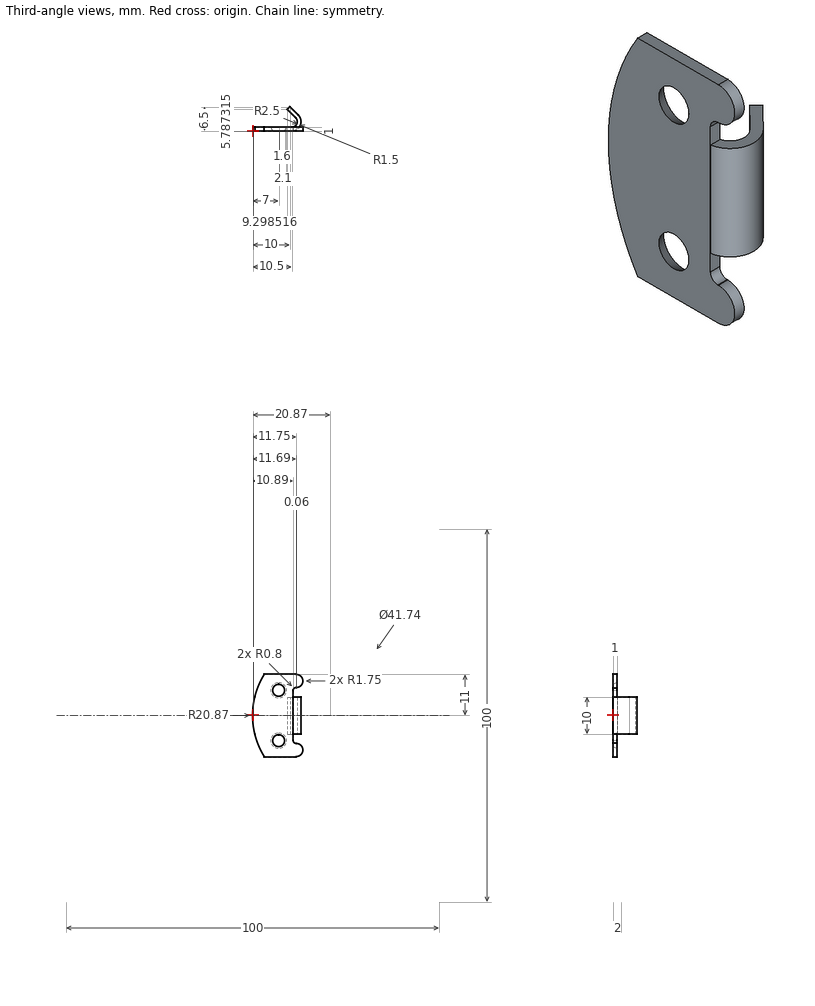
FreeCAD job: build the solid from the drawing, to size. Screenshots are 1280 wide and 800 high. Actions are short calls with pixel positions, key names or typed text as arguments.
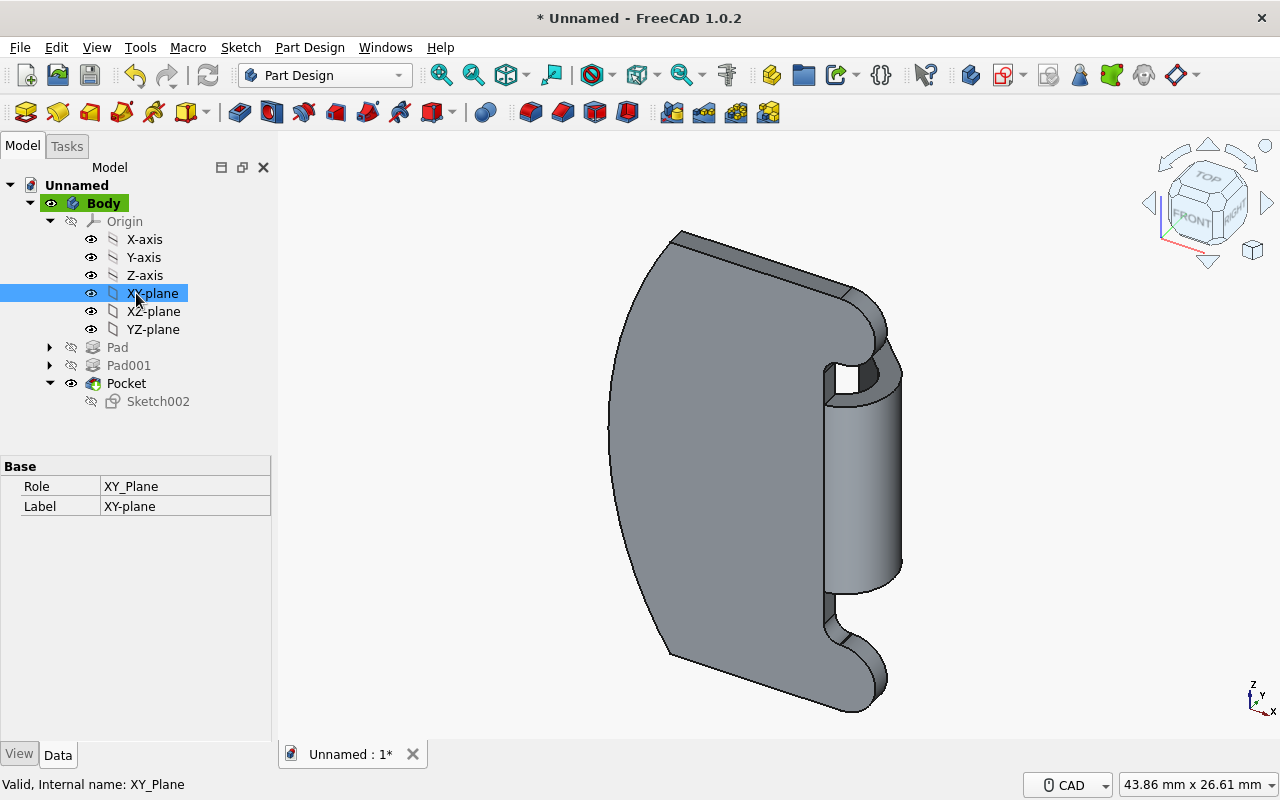
click(1176, 76)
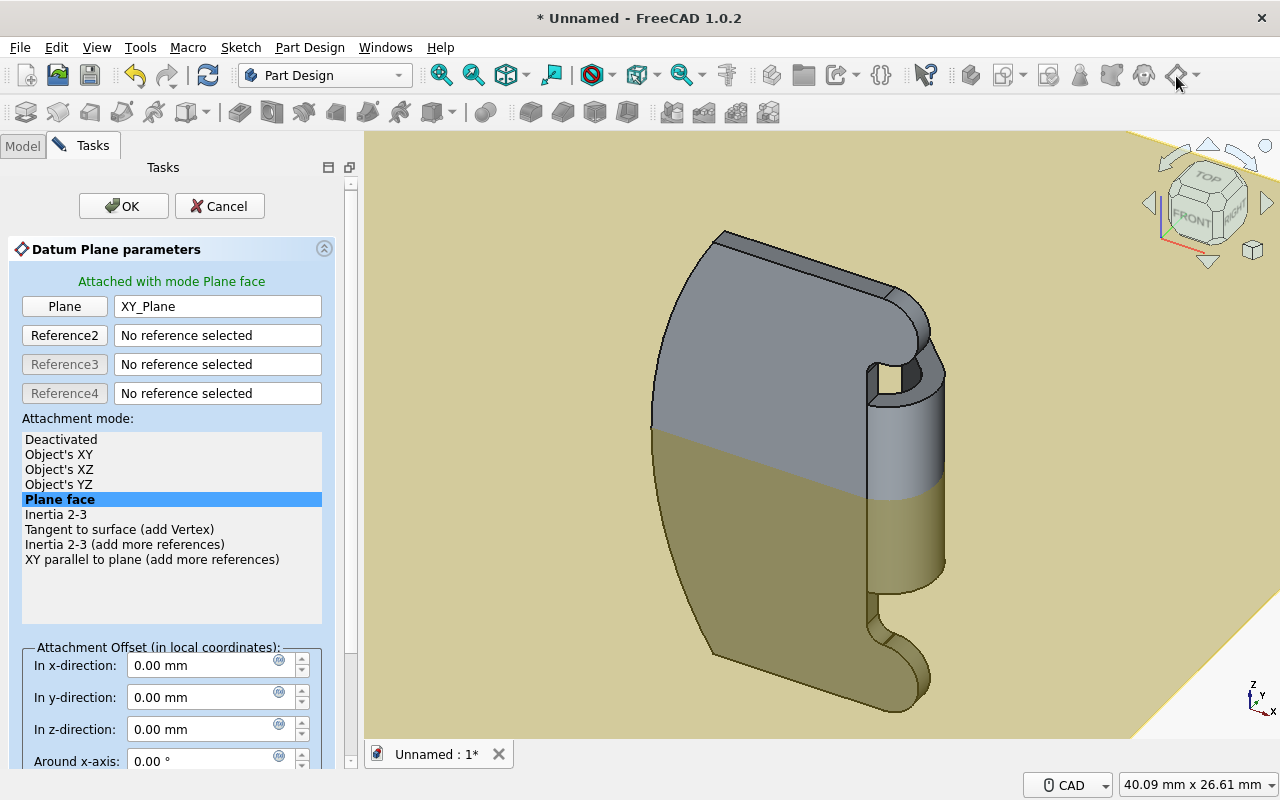
triple_click(210, 729)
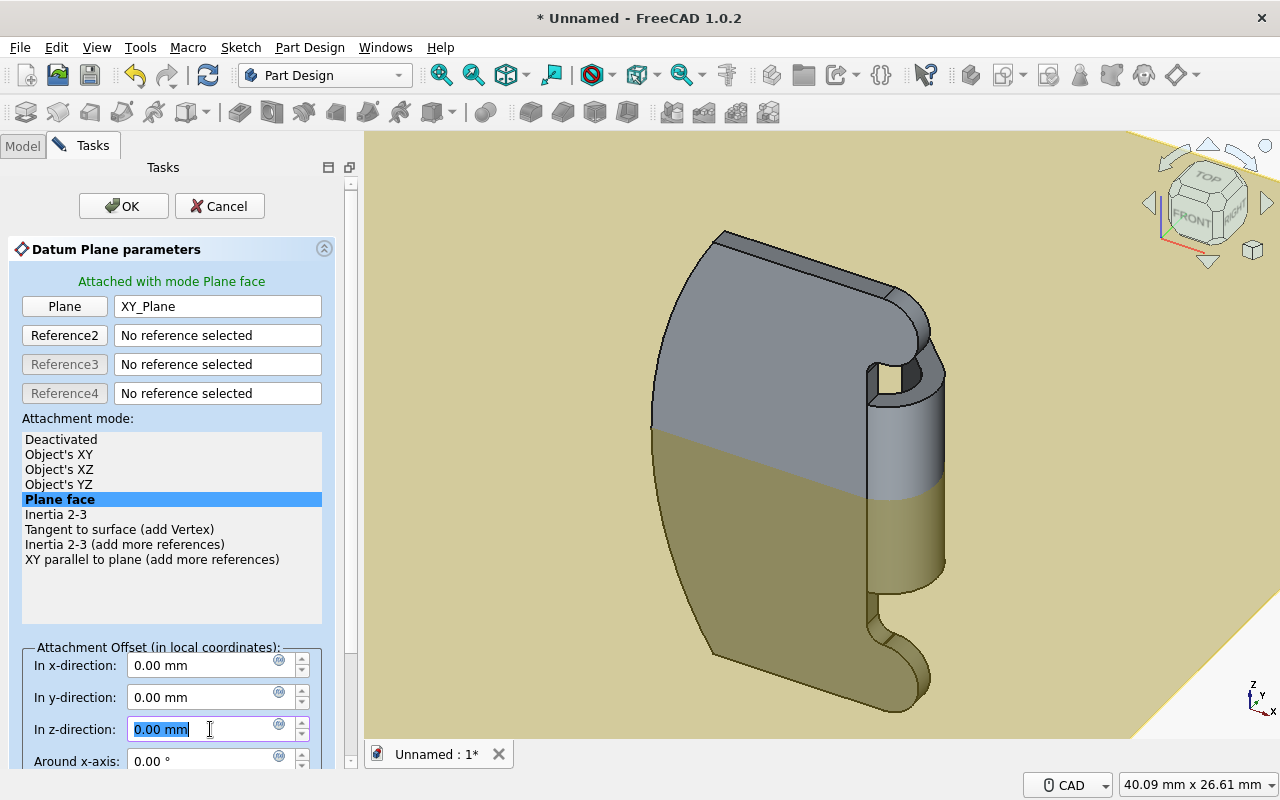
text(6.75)
key(Tab)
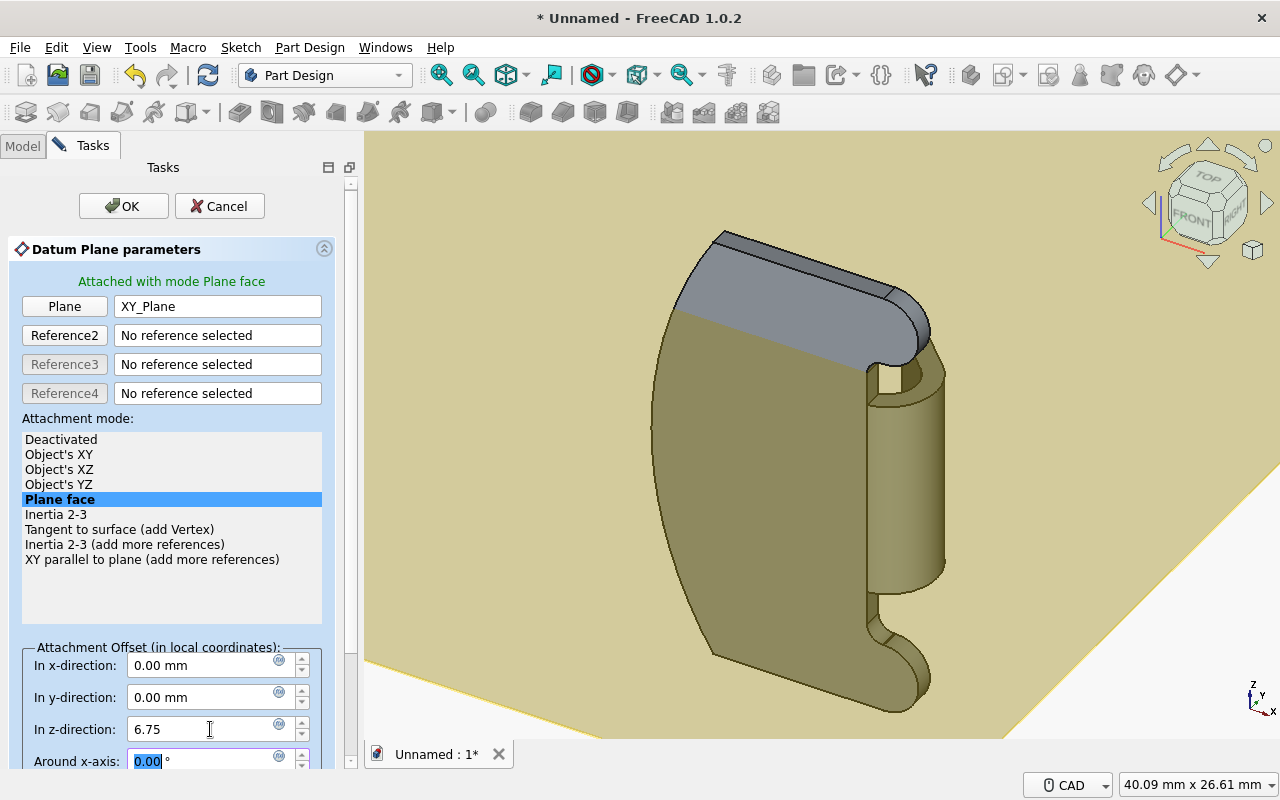
click(124, 206)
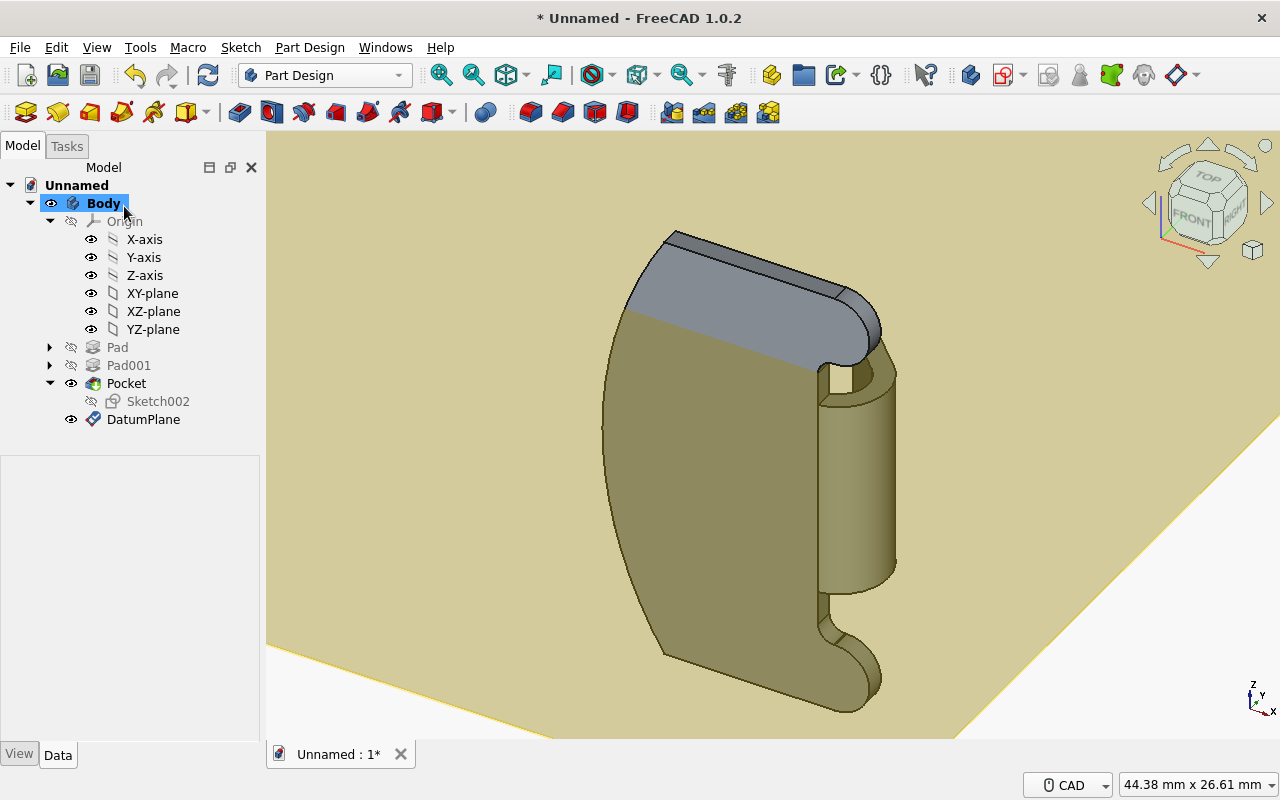
click(116, 419)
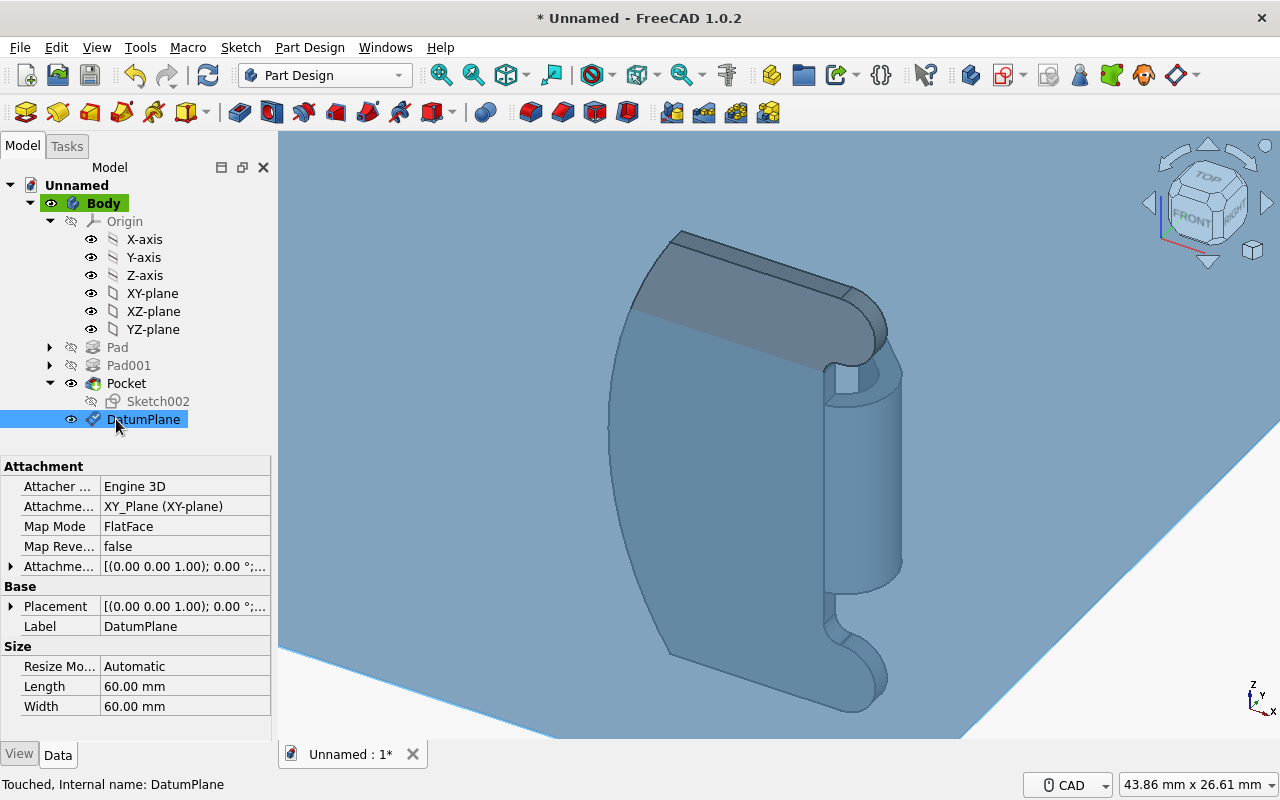
click(1004, 76)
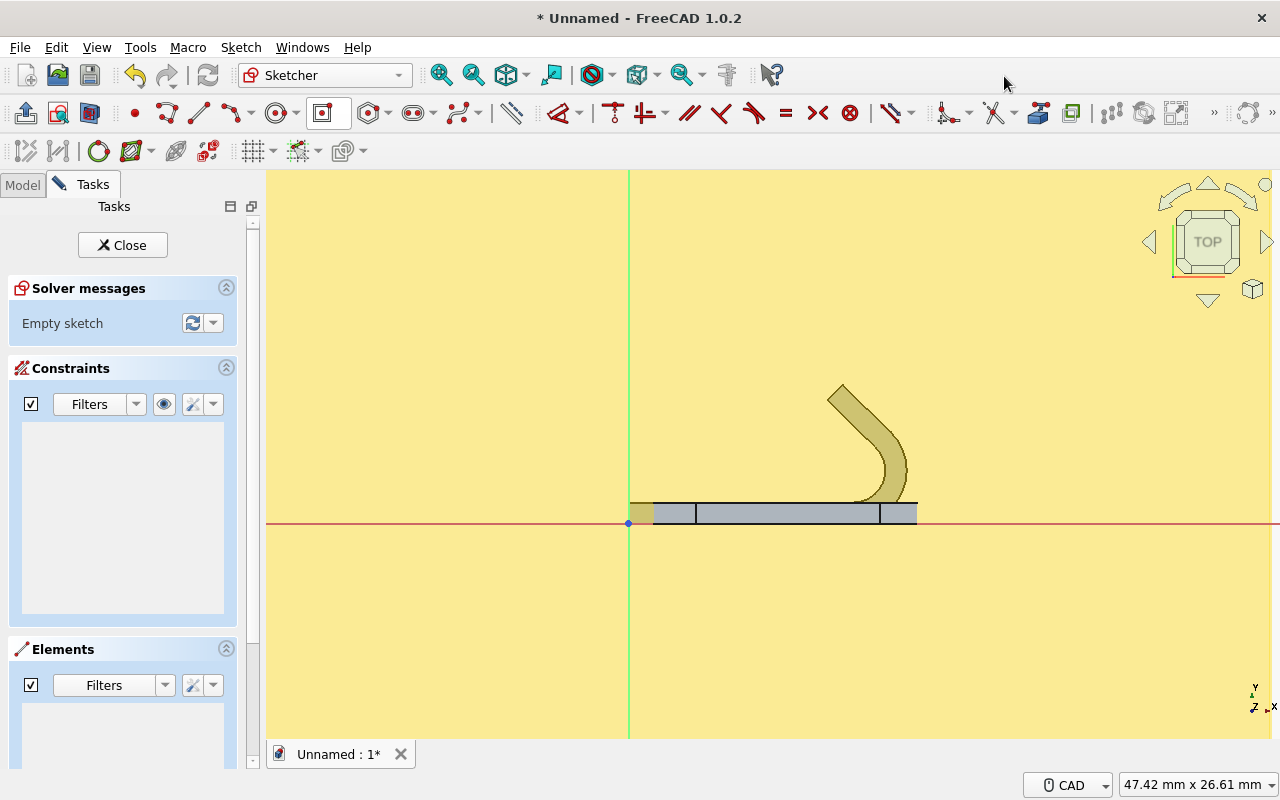
click(90, 114)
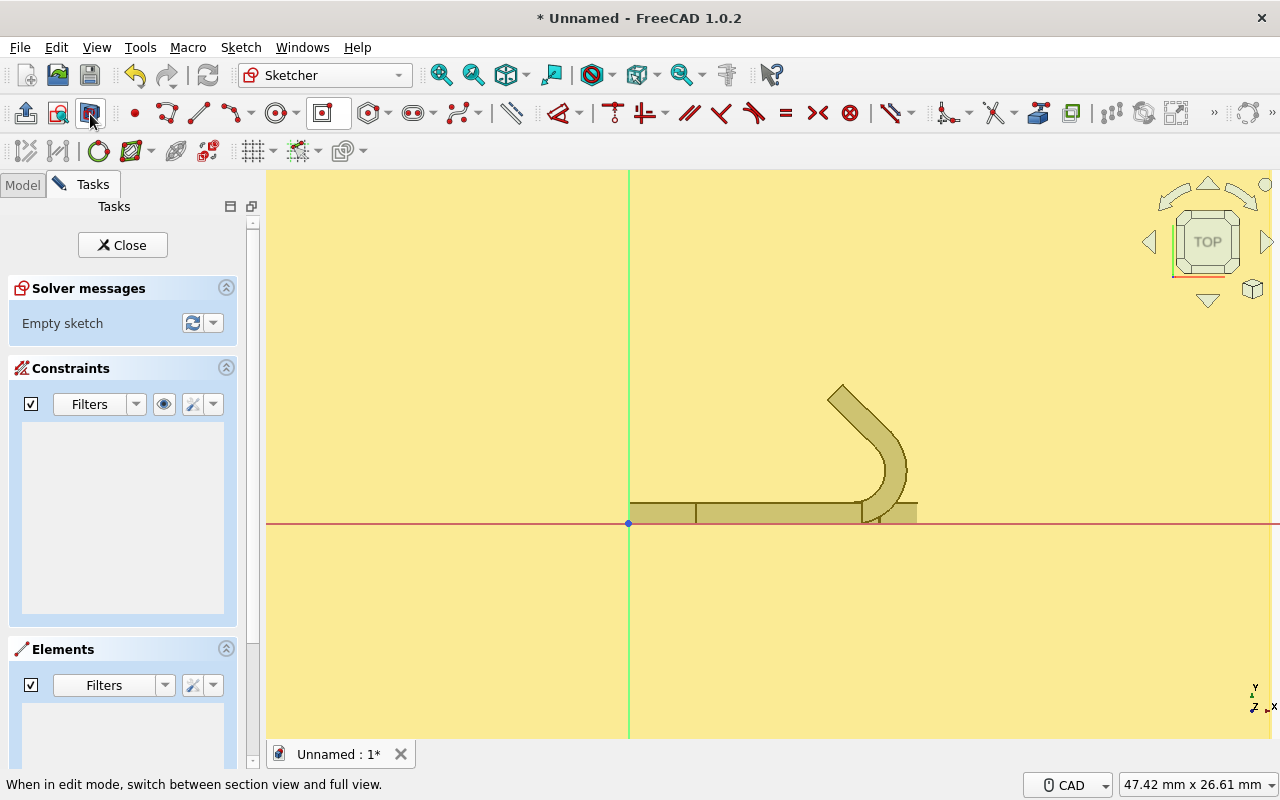
scroll(811, 514, up, 12)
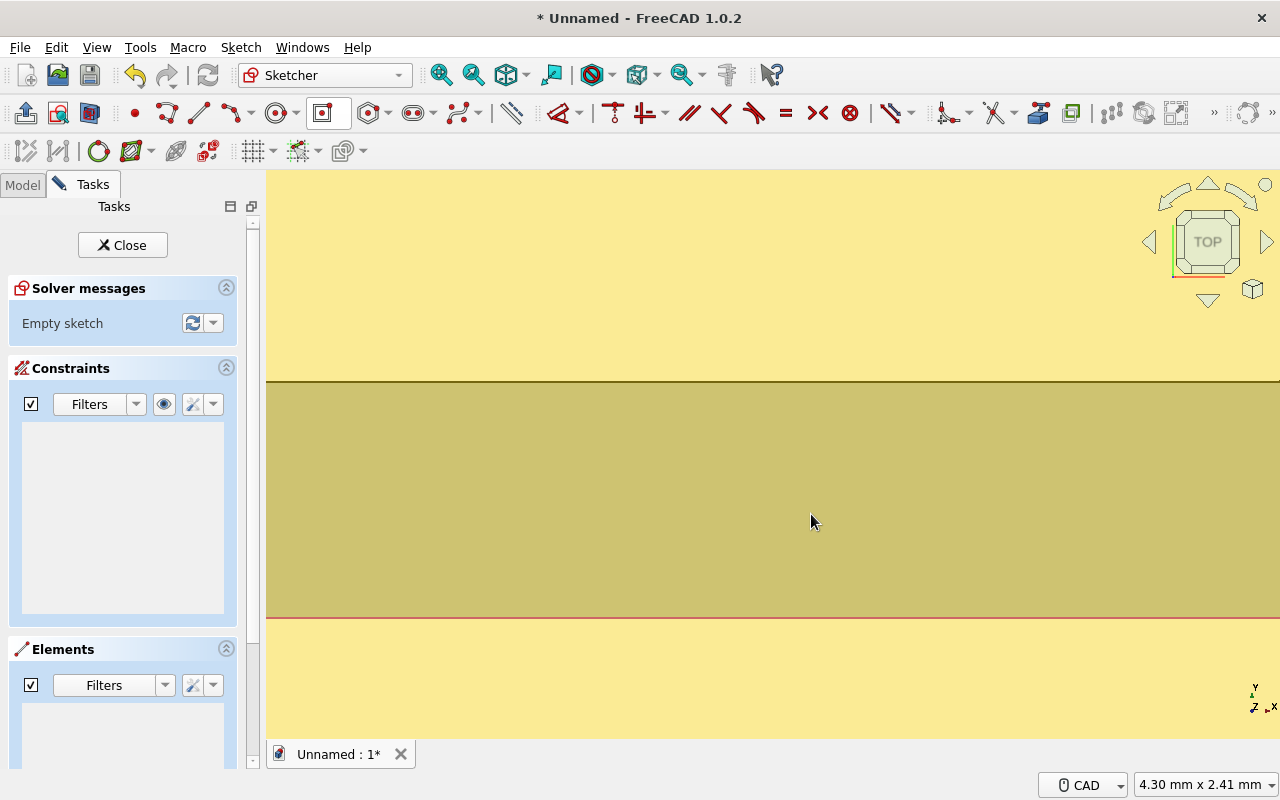
click(168, 114)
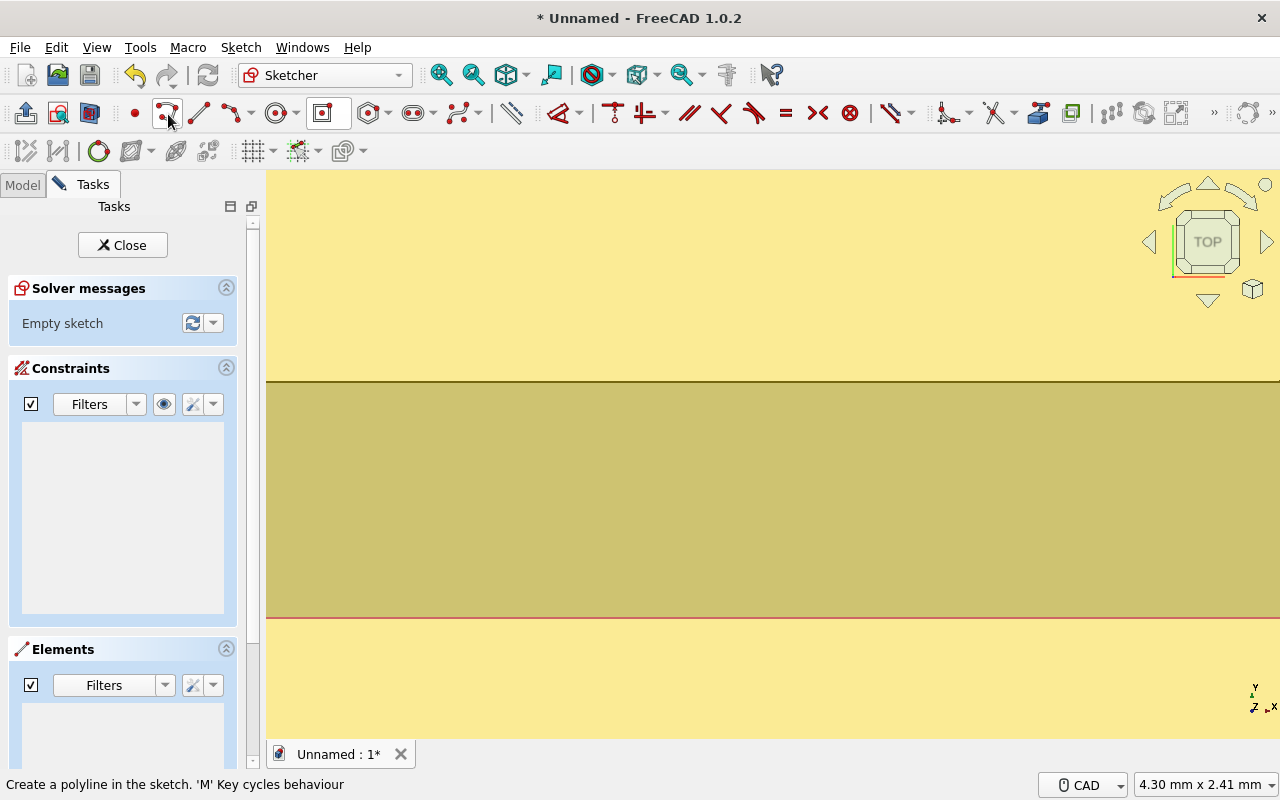
click(447, 618)
click(824, 609)
click(942, 382)
click(447, 382)
click(447, 618)